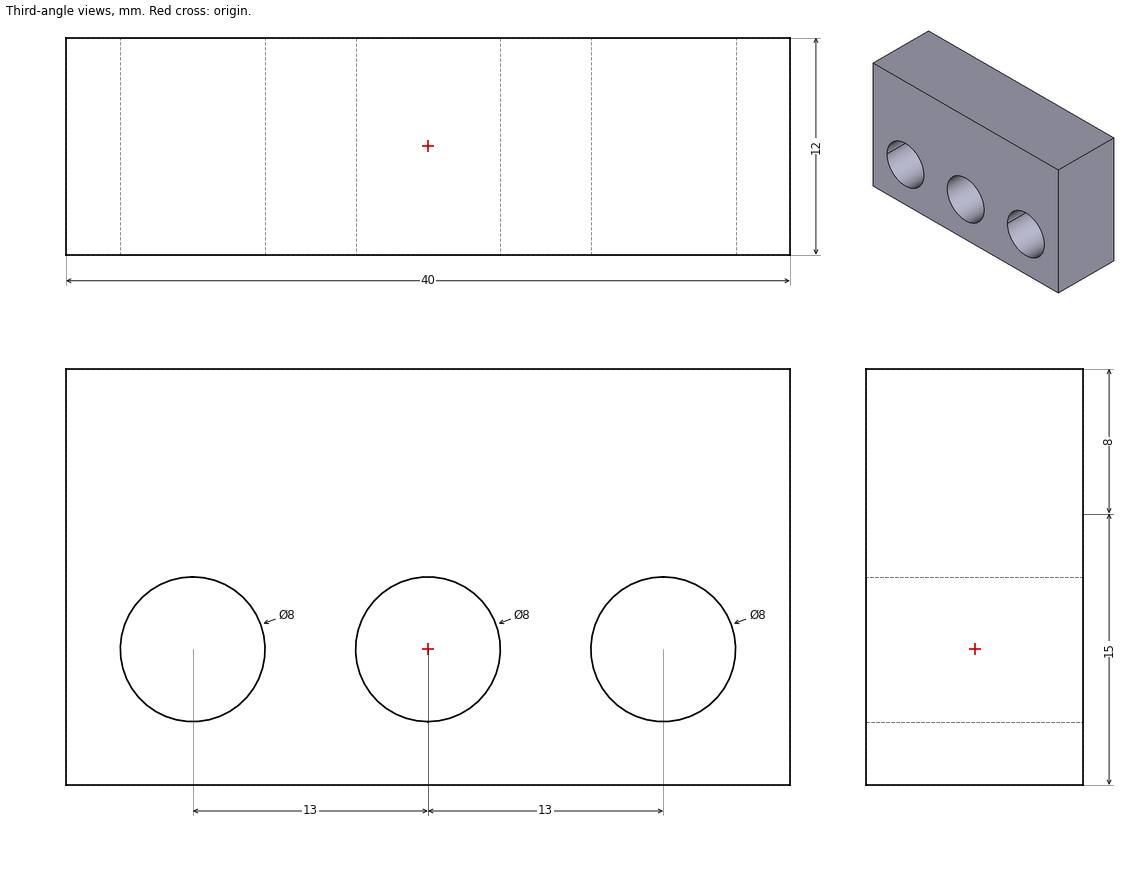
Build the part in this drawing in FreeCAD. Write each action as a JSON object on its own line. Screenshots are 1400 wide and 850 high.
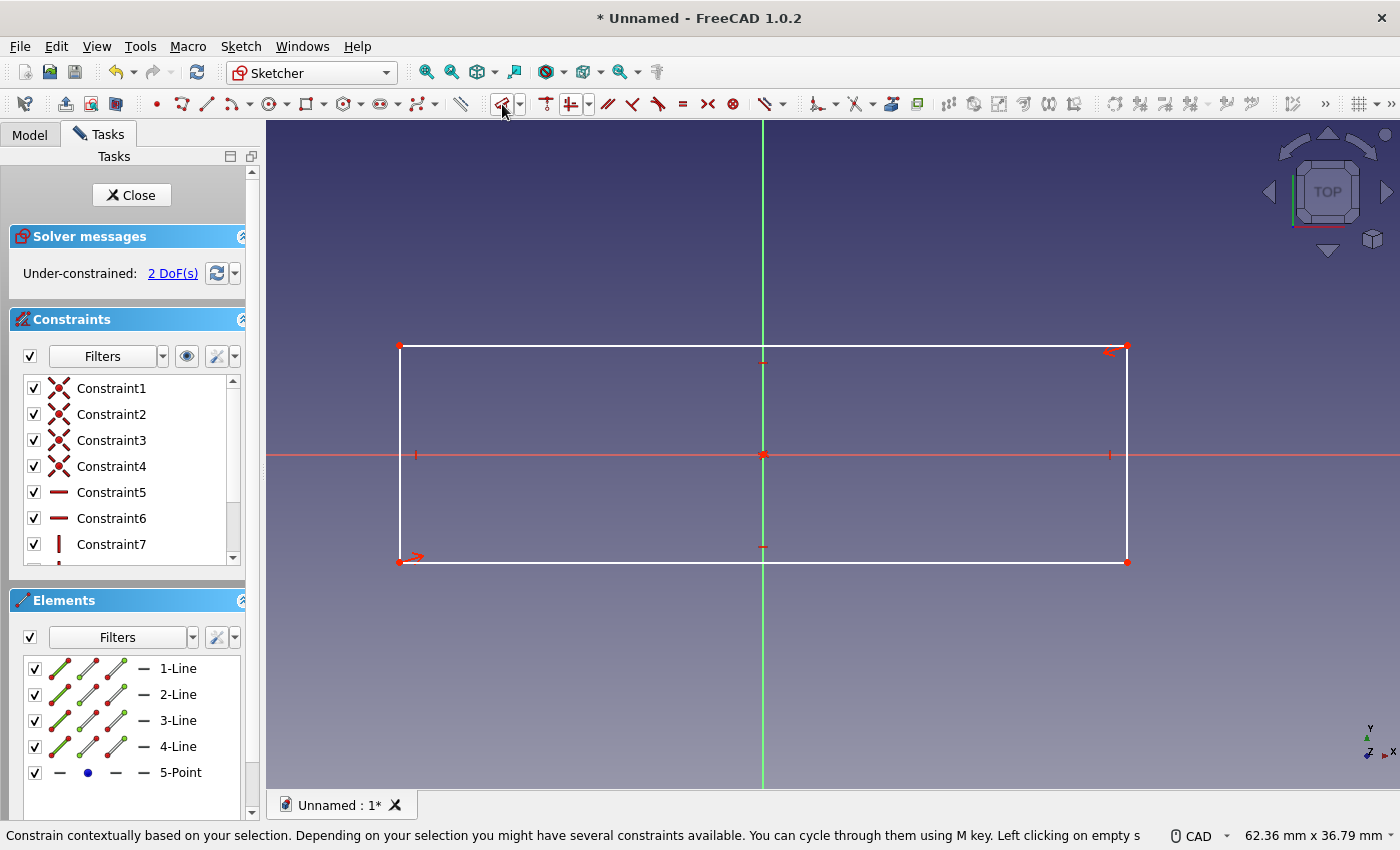
{"action": "left_click", "coordinate": [618, 563]}
{"action": "left_click", "coordinate": [596, 597]}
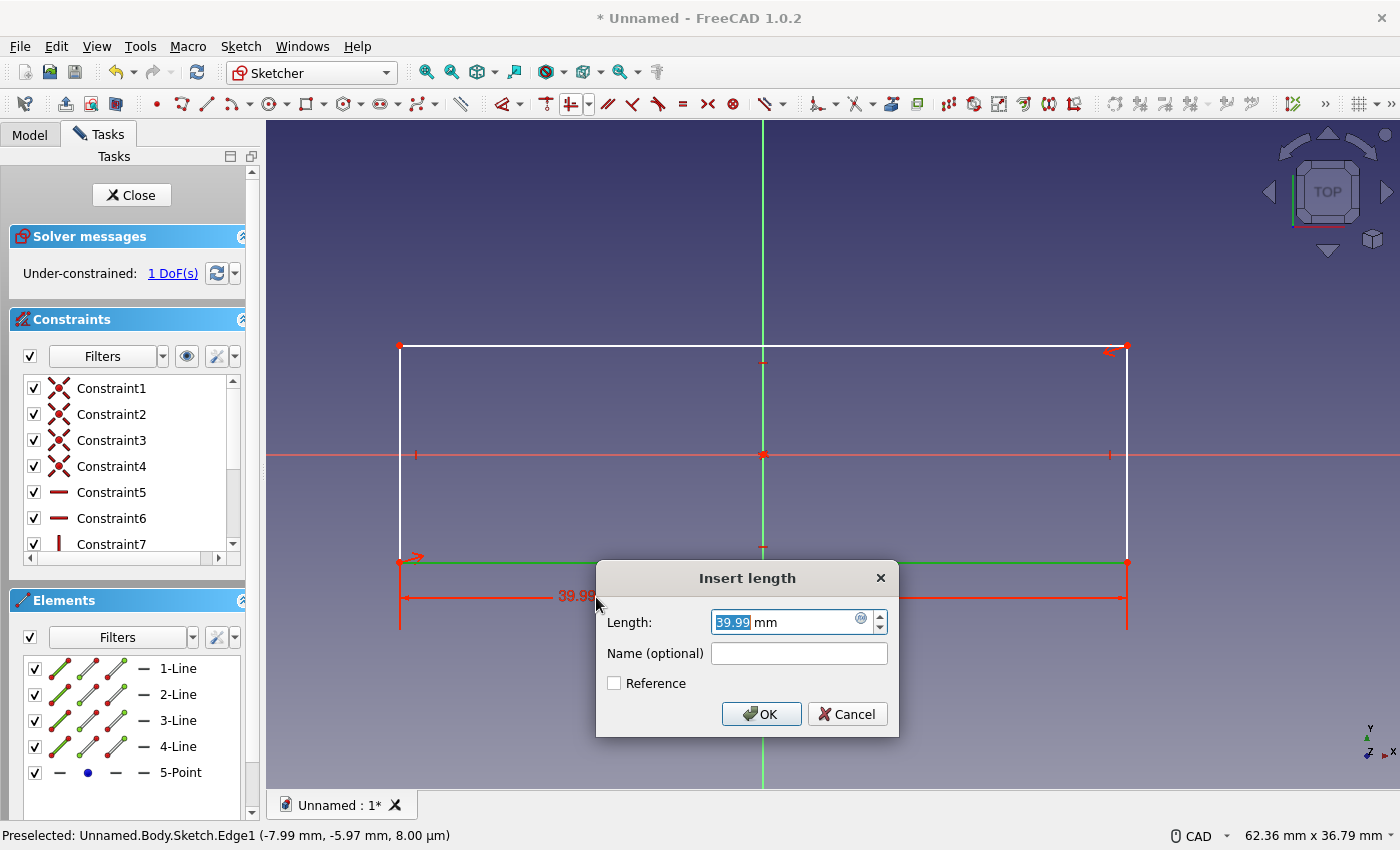
{"action": "type", "text": "40"}
{"action": "key", "text": "Return"}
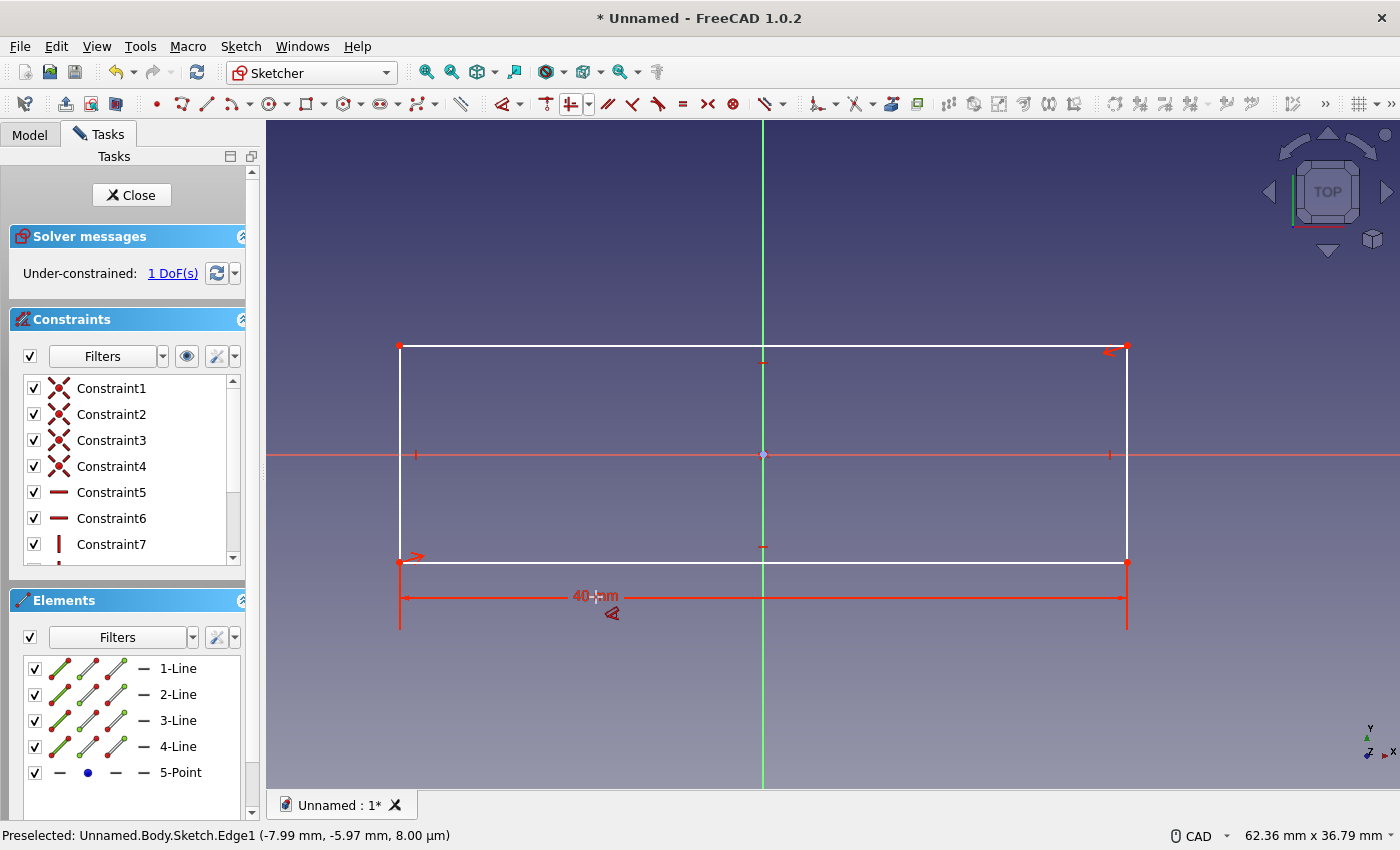
{"action": "left_click", "coordinate": [1127, 498]}
{"action": "left_click", "coordinate": [1161, 405]}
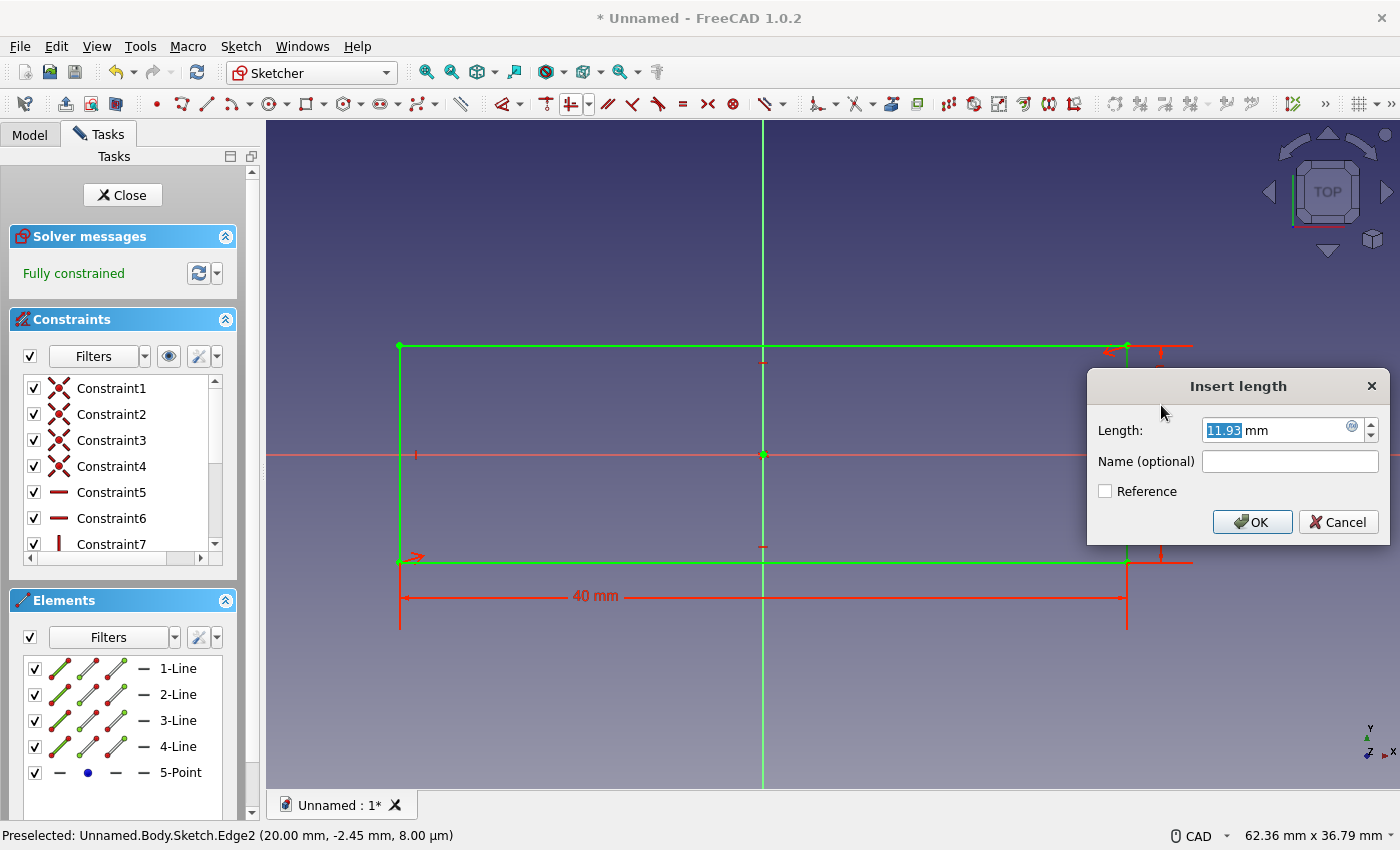
{"action": "type", "text": "12"}
{"action": "key", "text": "Return"}
{"action": "key", "text": "Escape"}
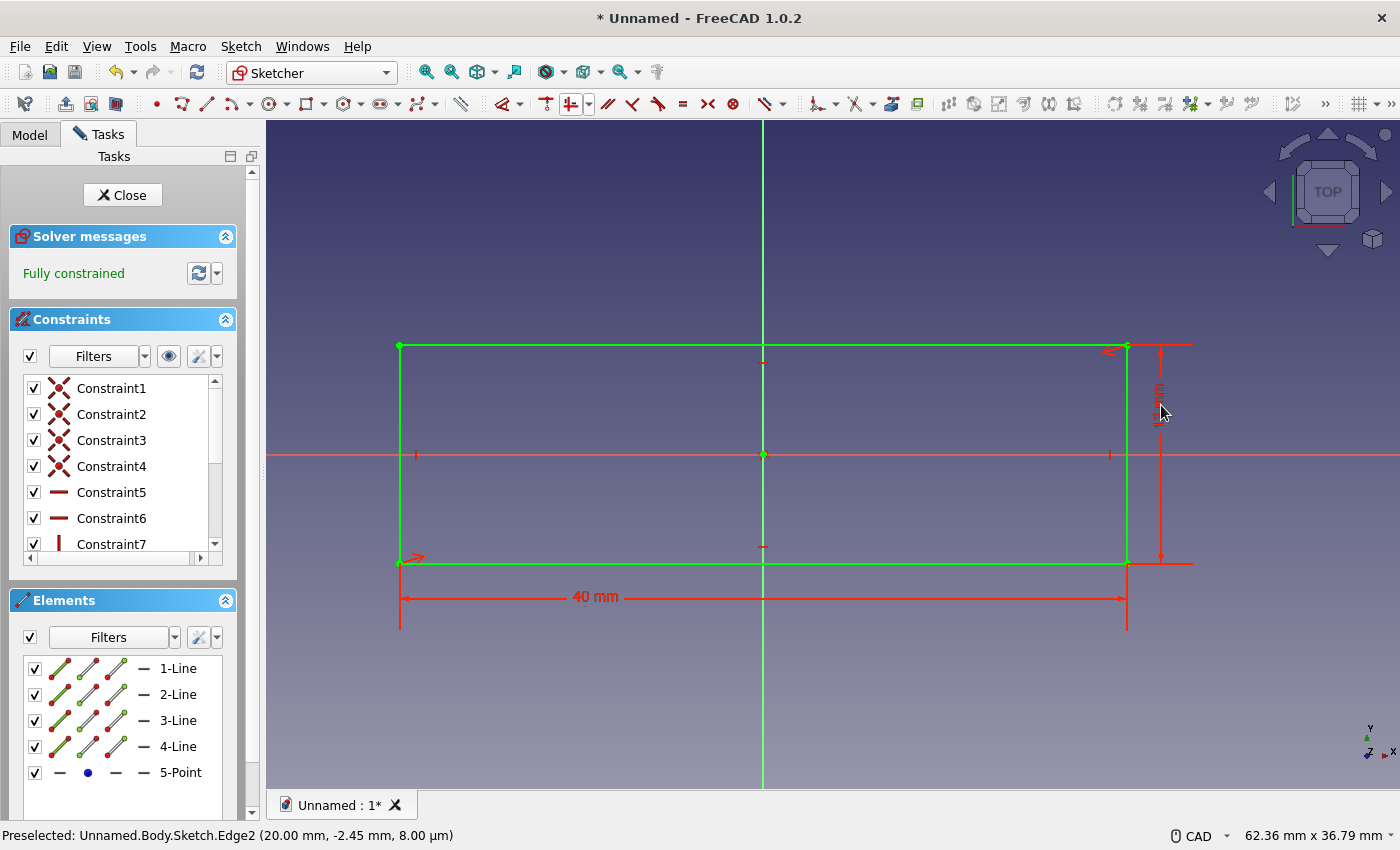
{"action": "left_click", "coordinate": [123, 195]}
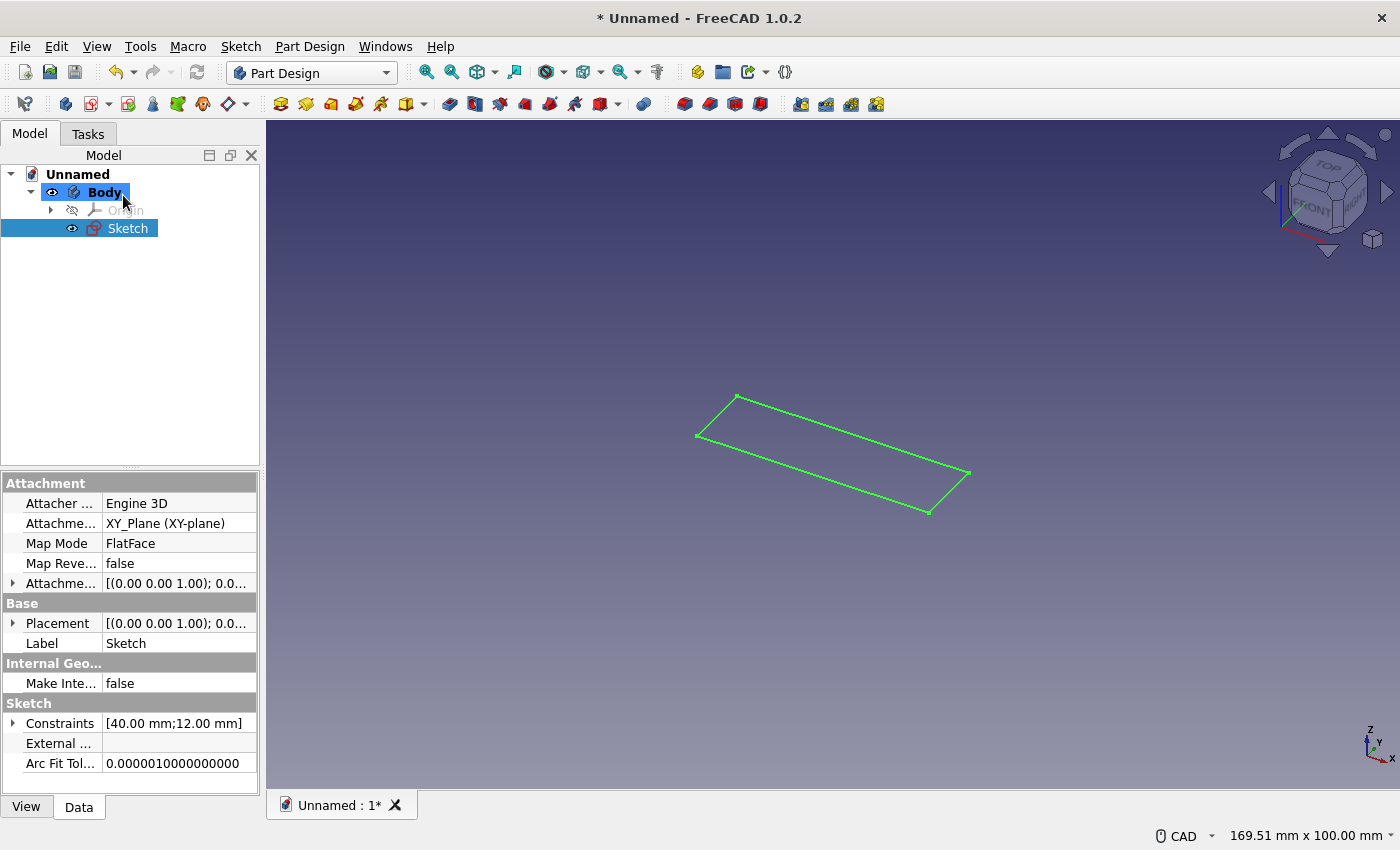
{"action": "left_click", "coordinate": [281, 104]}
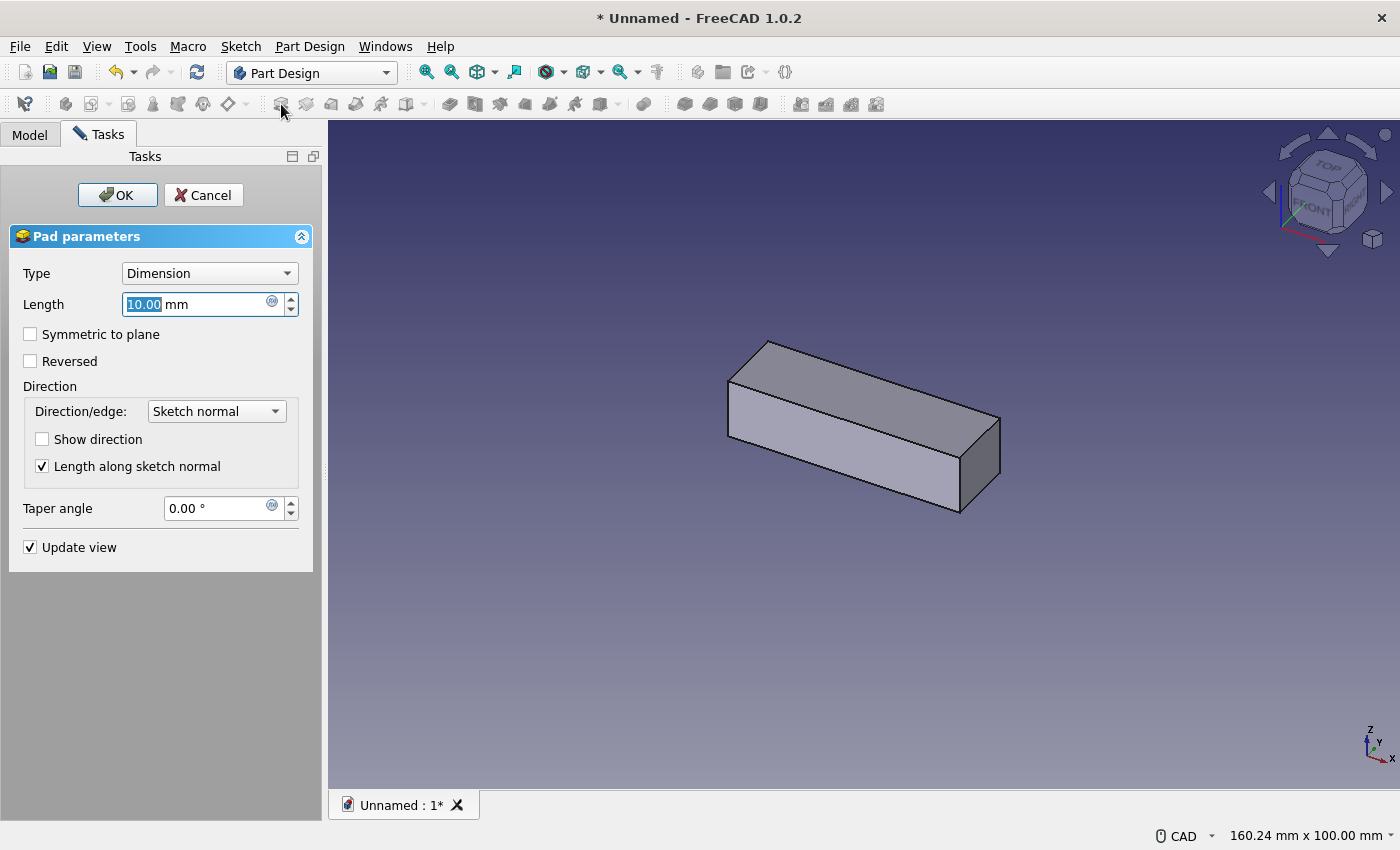
{"action": "type", "text": "15"}
{"action": "key", "text": "Tab"}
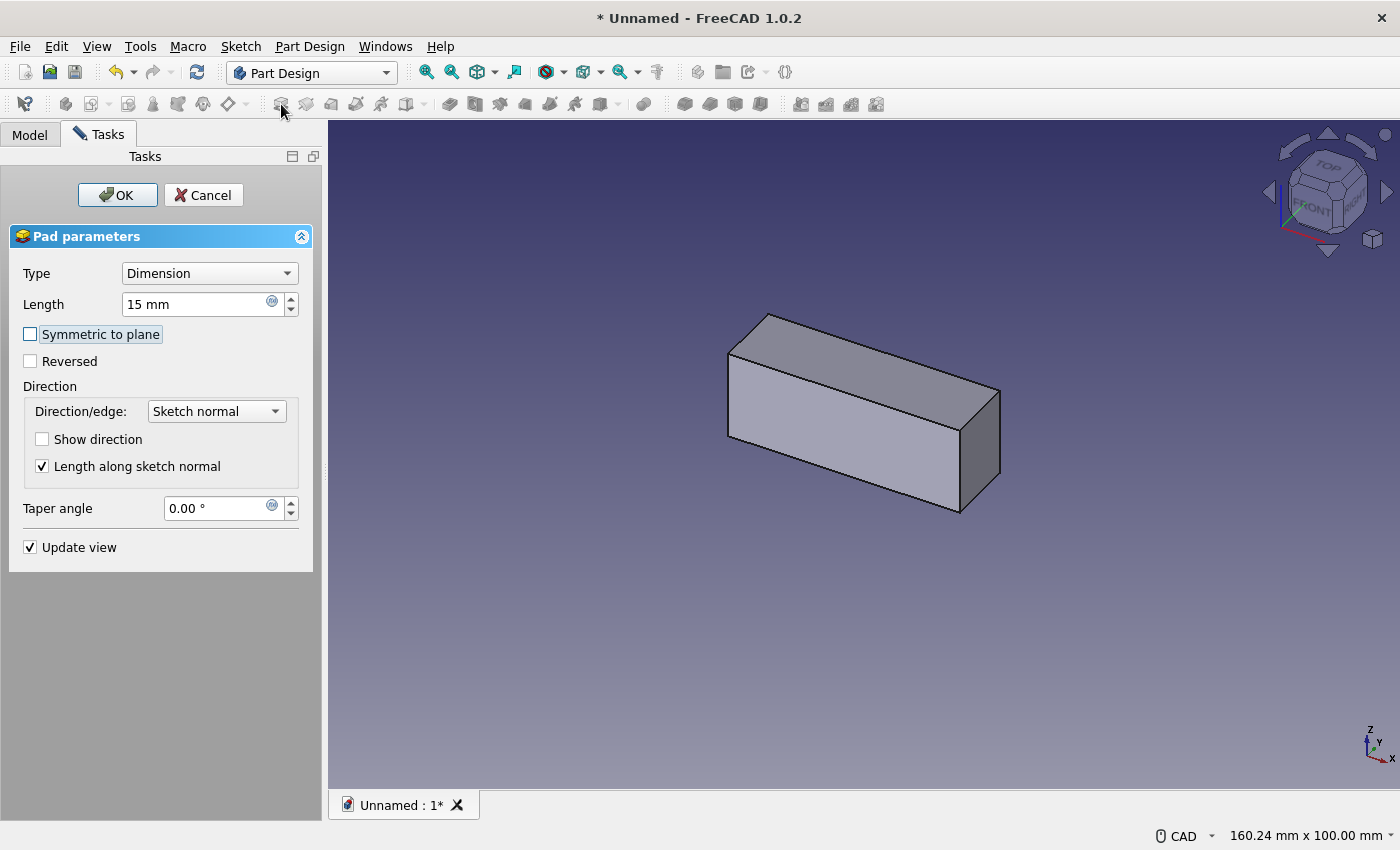
{"action": "left_click", "coordinate": [31, 334]}